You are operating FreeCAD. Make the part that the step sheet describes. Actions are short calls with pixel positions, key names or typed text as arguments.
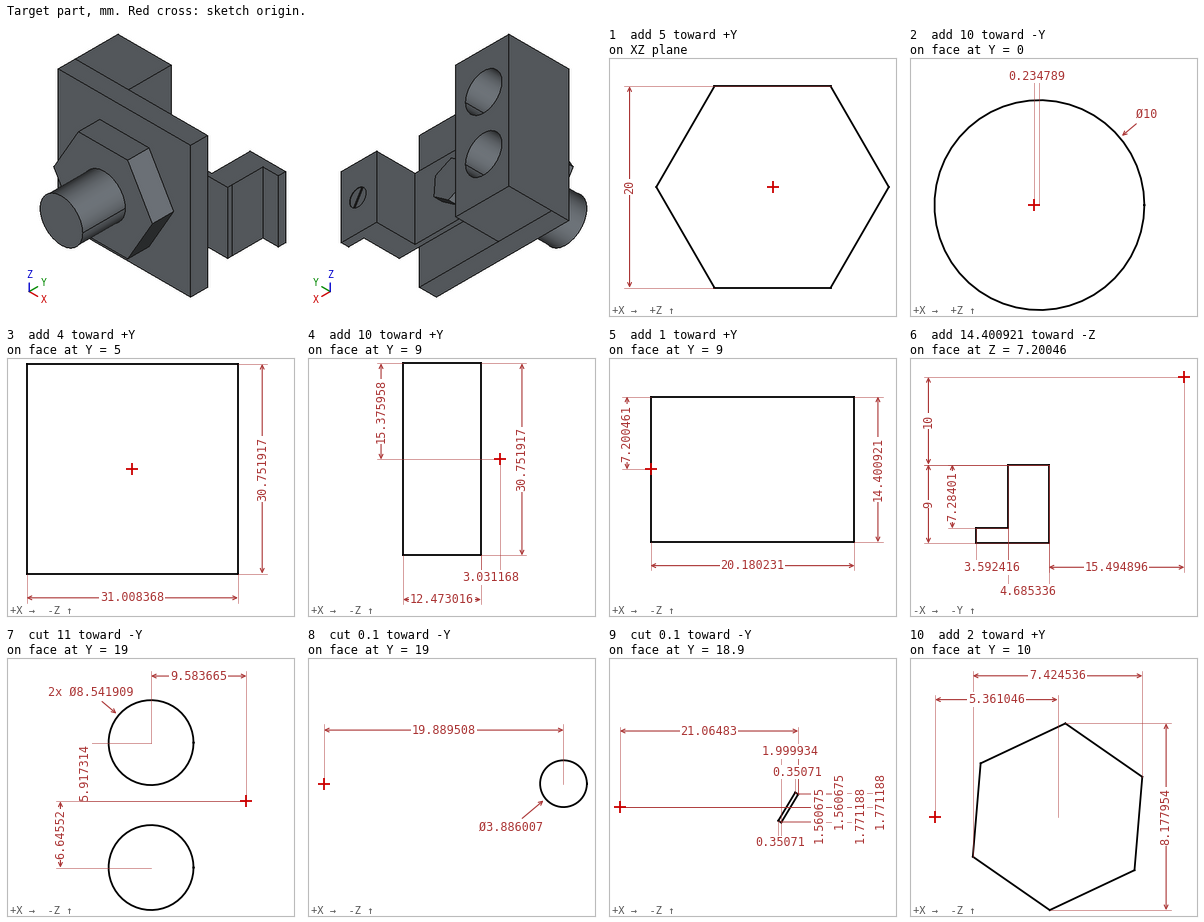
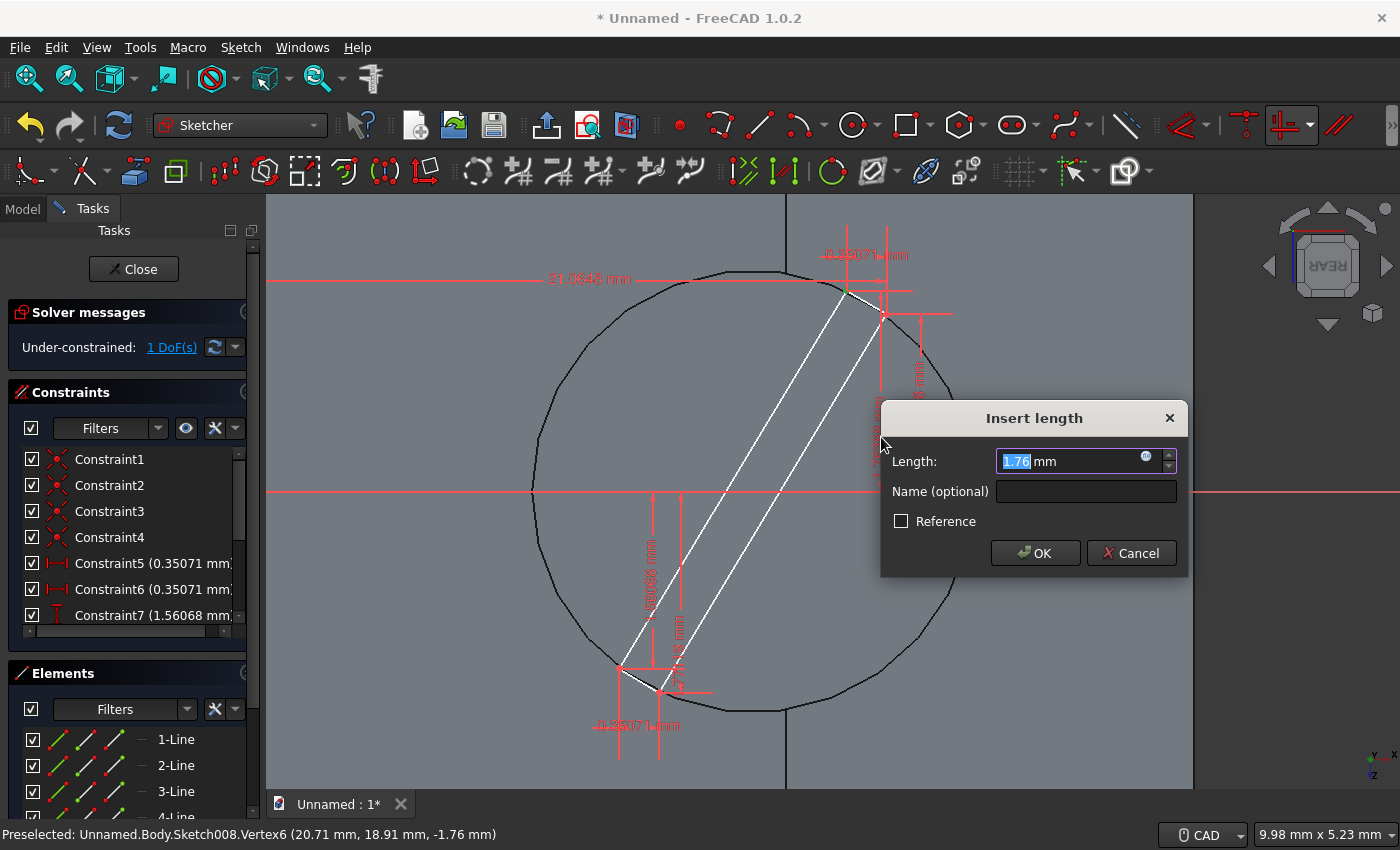
text(1.771188)
key(Return)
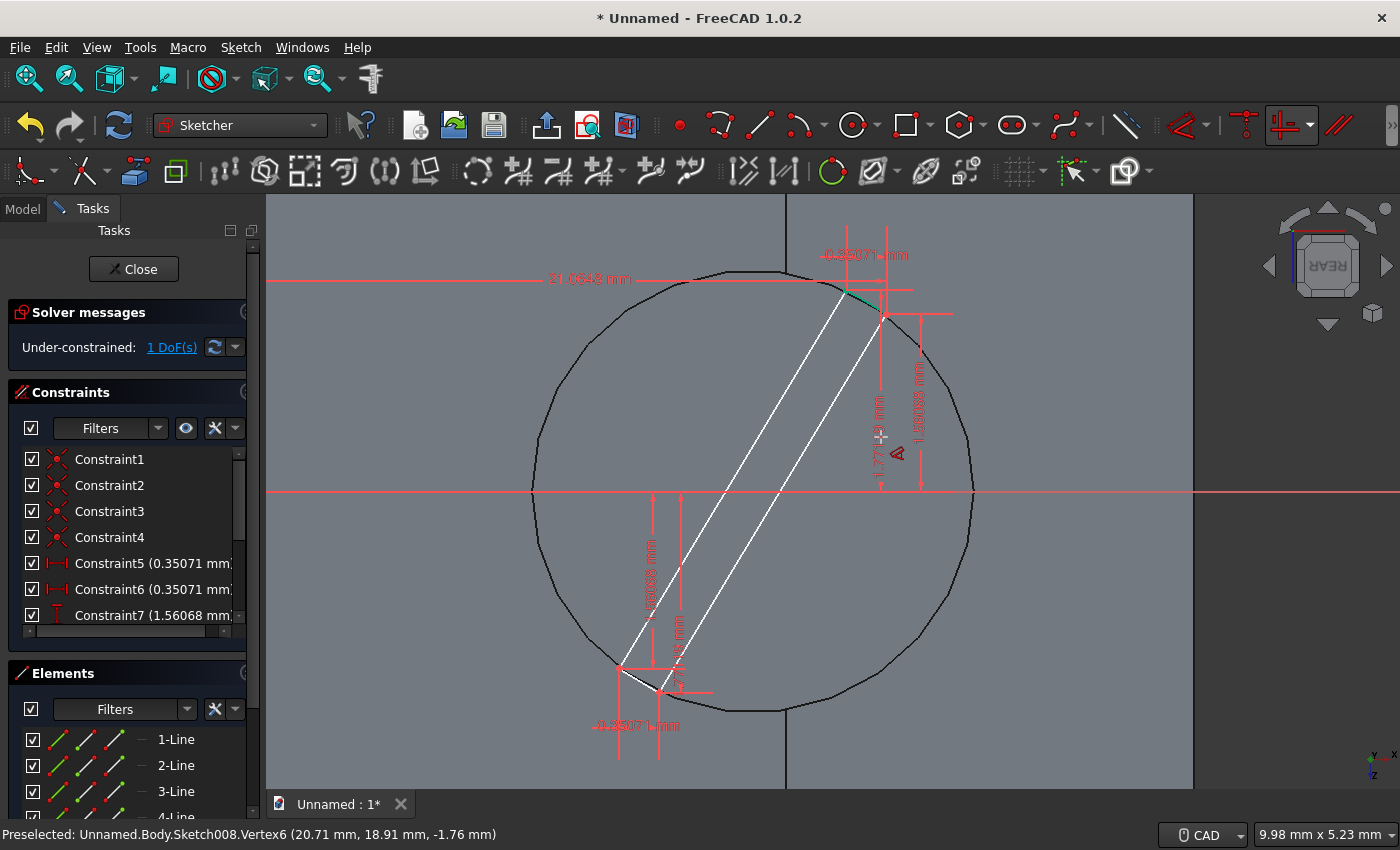
click(727, 579)
click(773, 727)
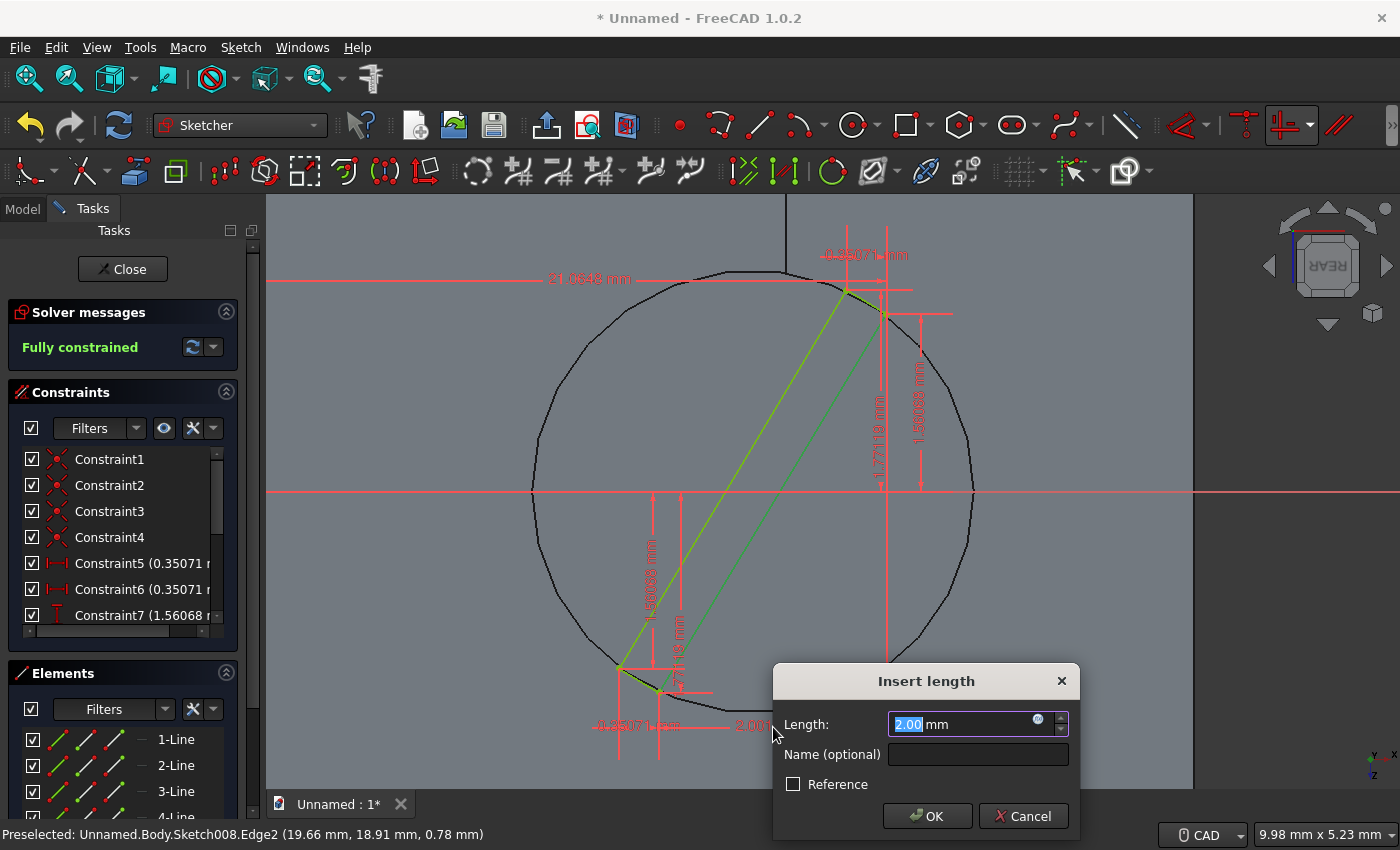
text(1.999934)
key(Return)
key(Escape)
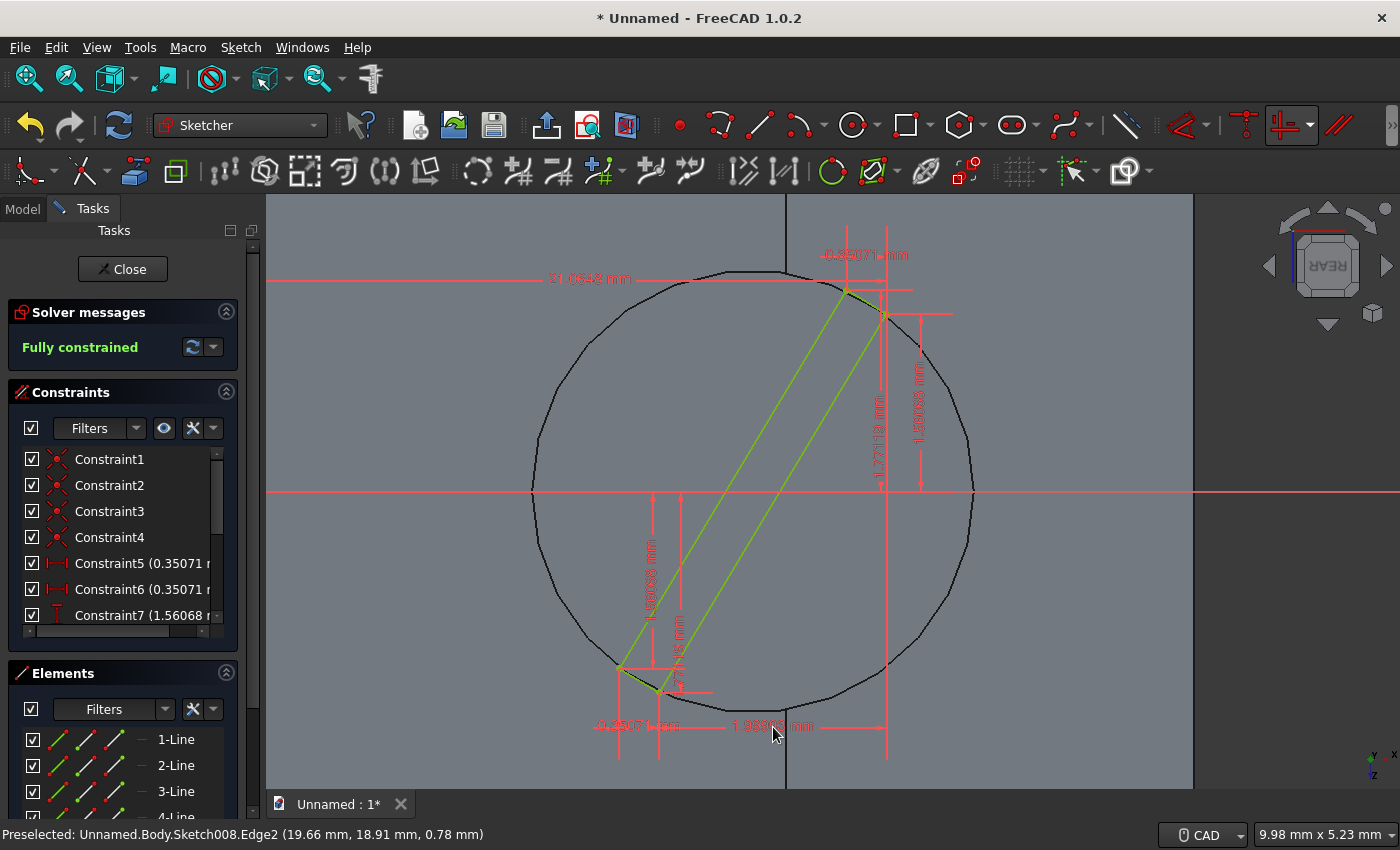
click(123, 269)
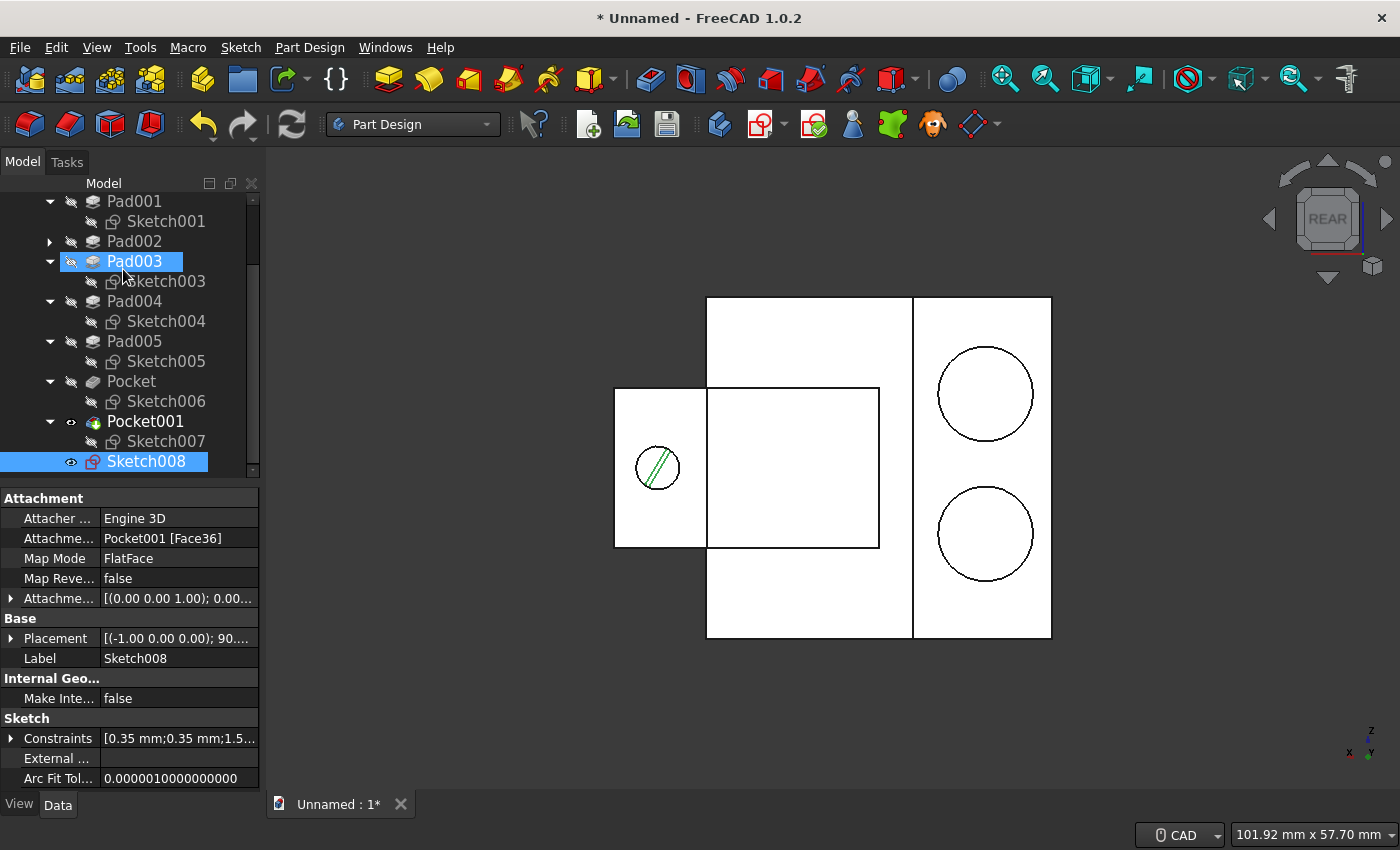
click(652, 80)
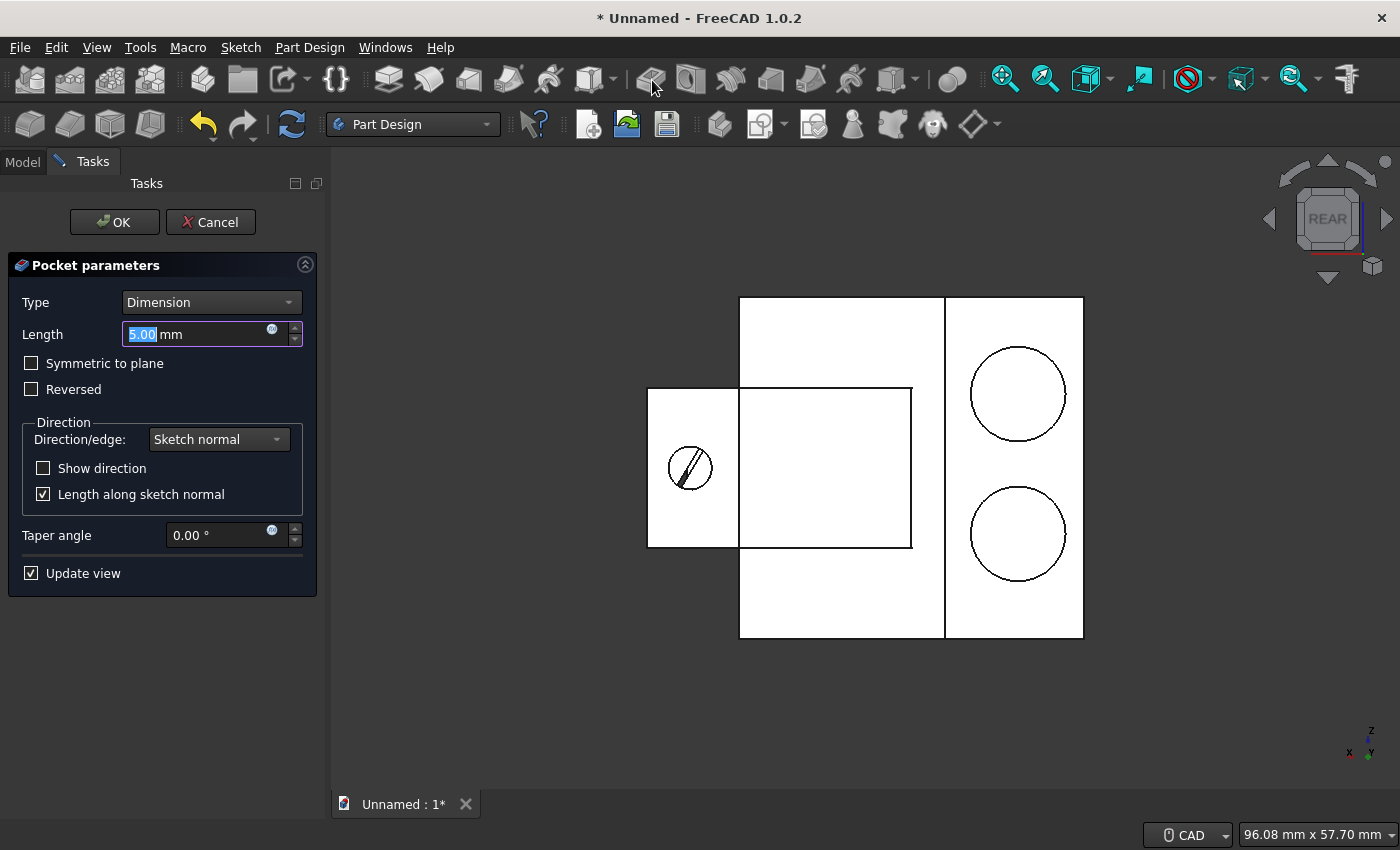
text(0.1)
key(Tab)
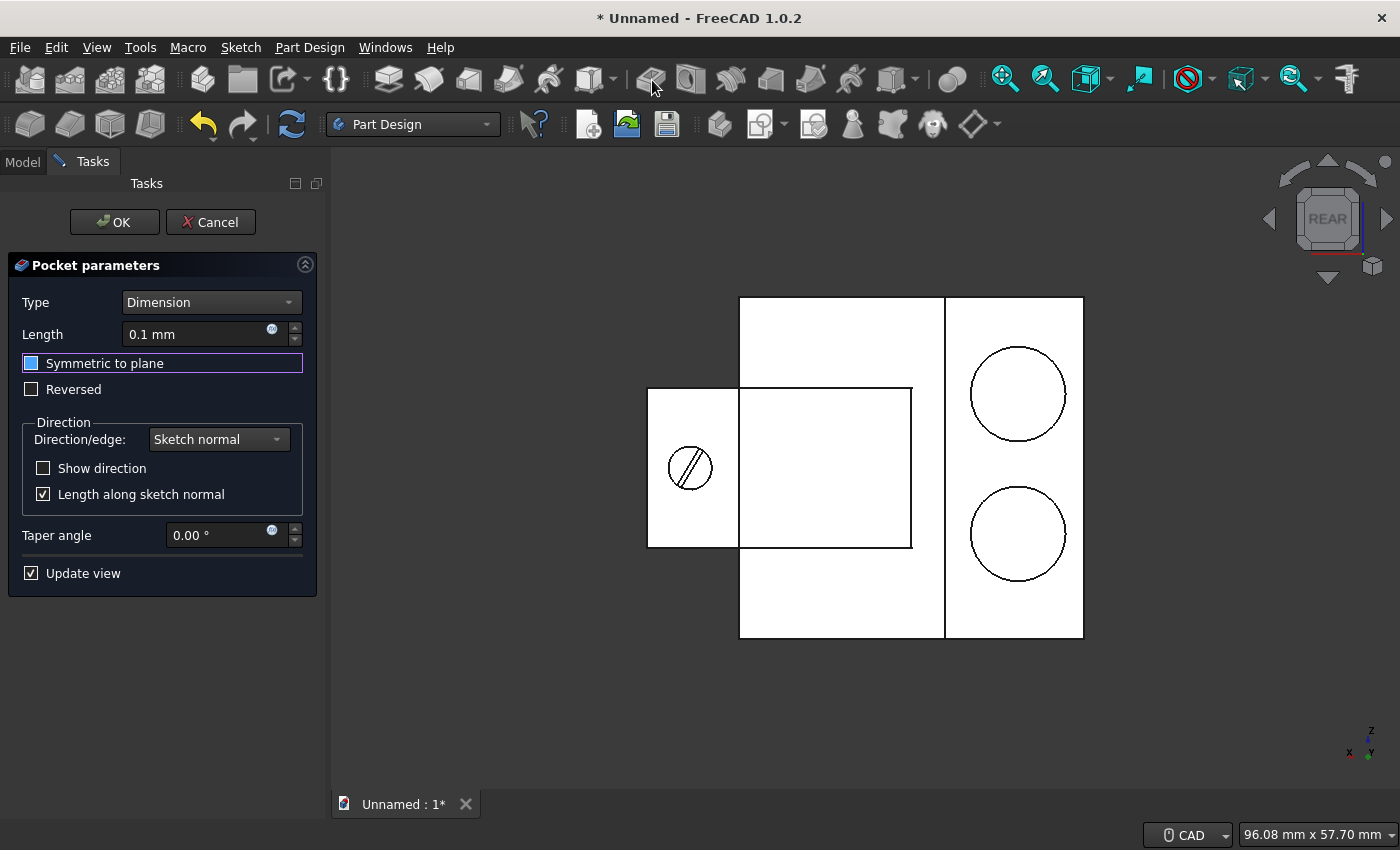
click(115, 222)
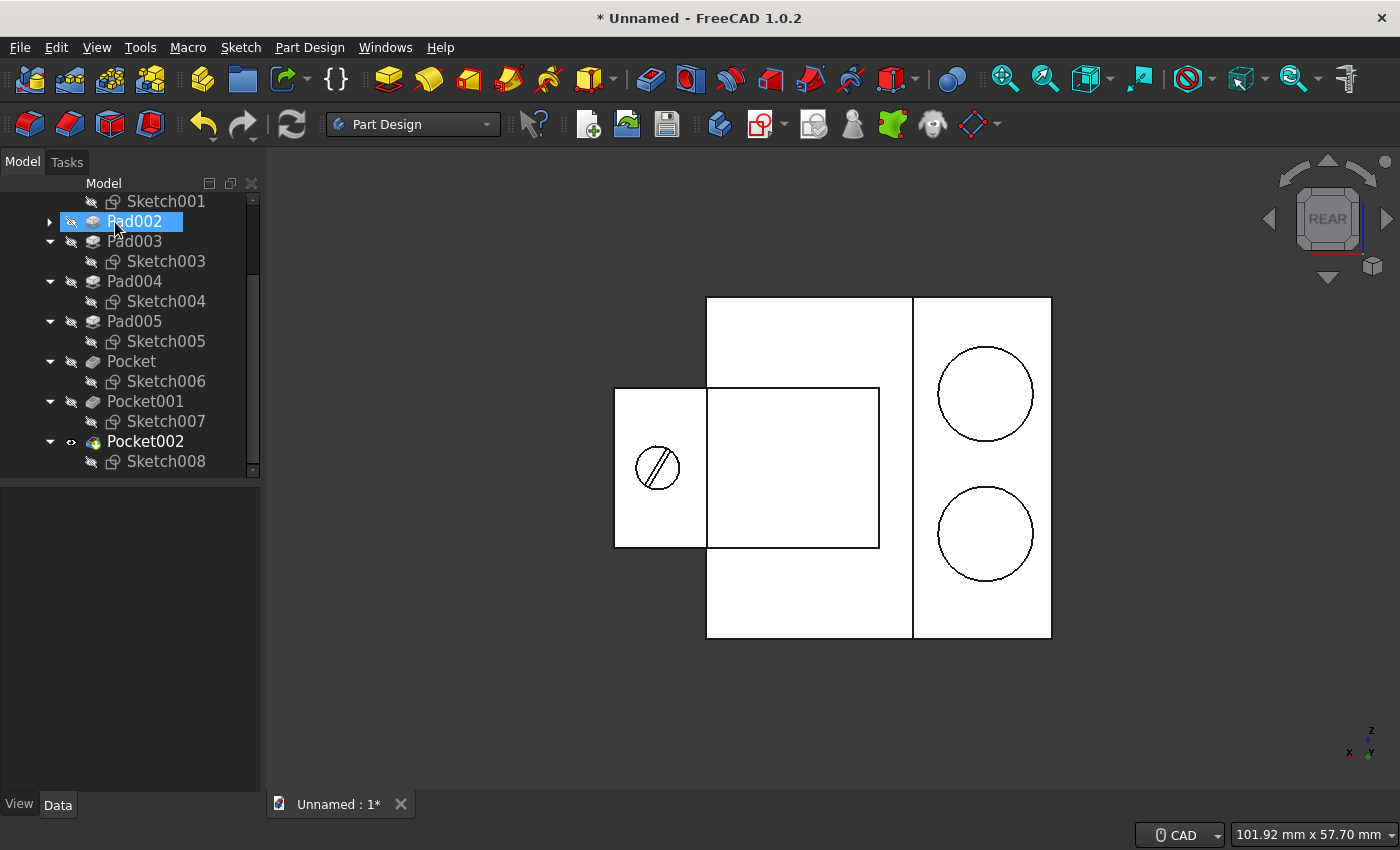
click(793, 467)